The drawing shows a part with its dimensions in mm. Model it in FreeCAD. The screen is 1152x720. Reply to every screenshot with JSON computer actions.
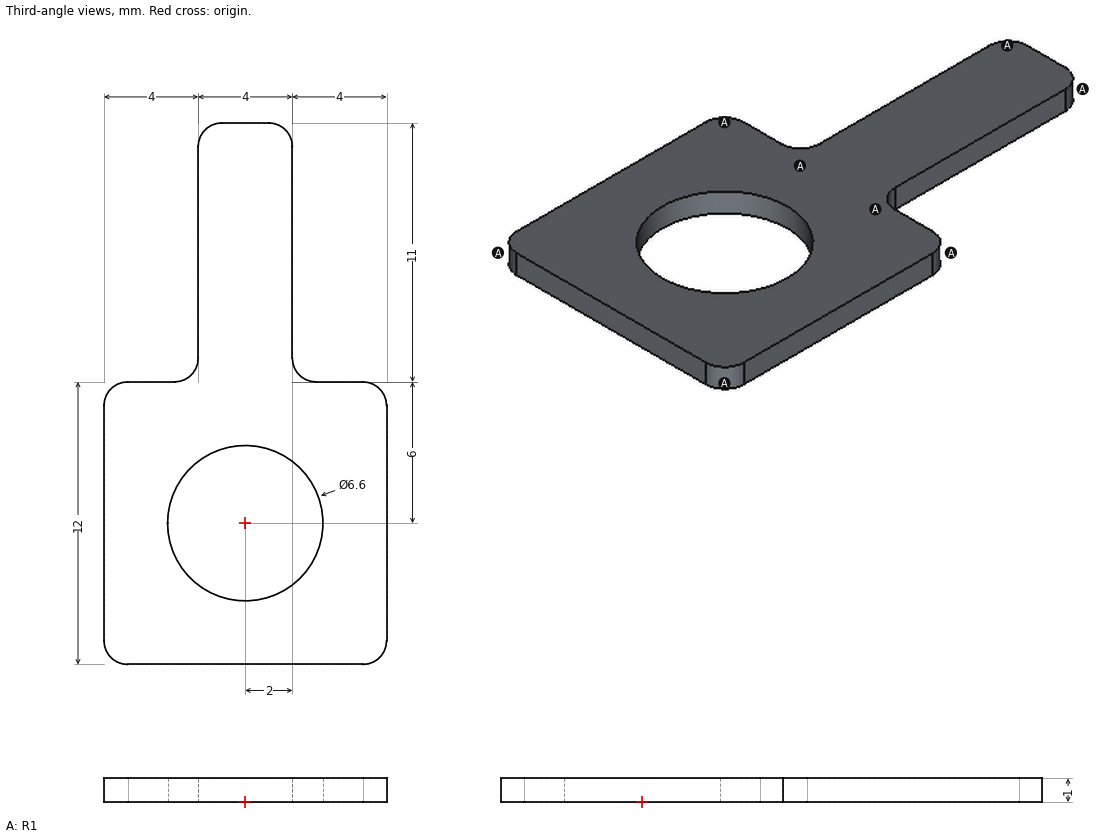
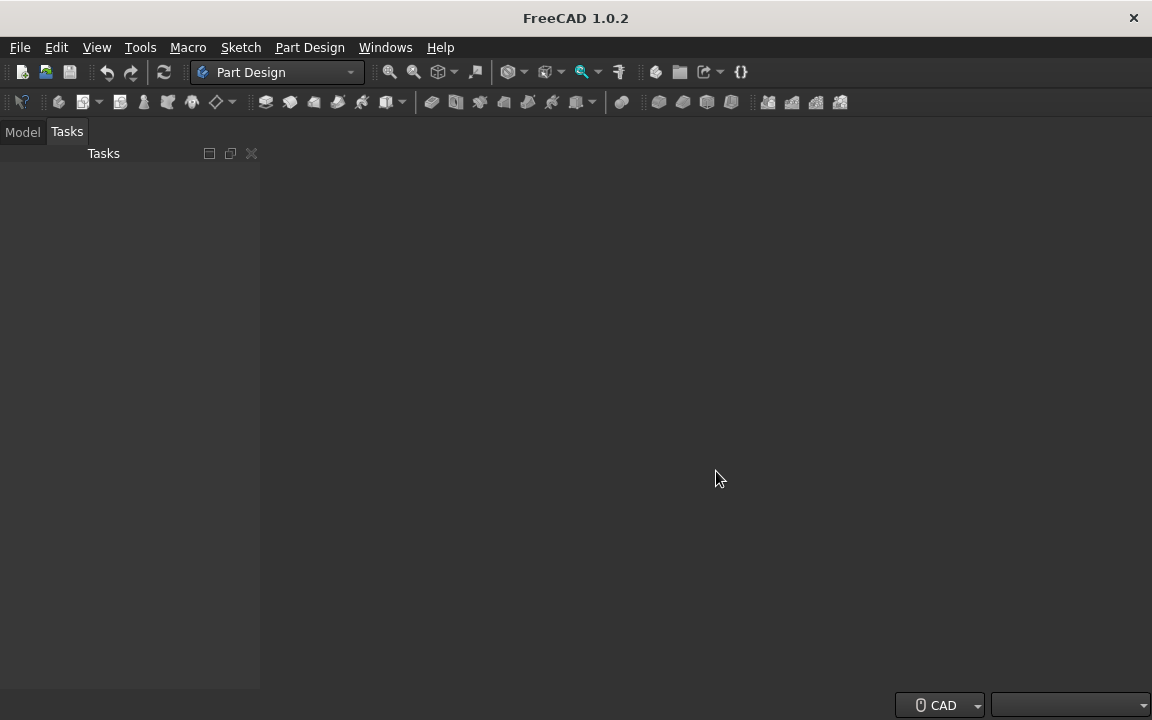
{"action": "left_click", "coordinate": [22, 72]}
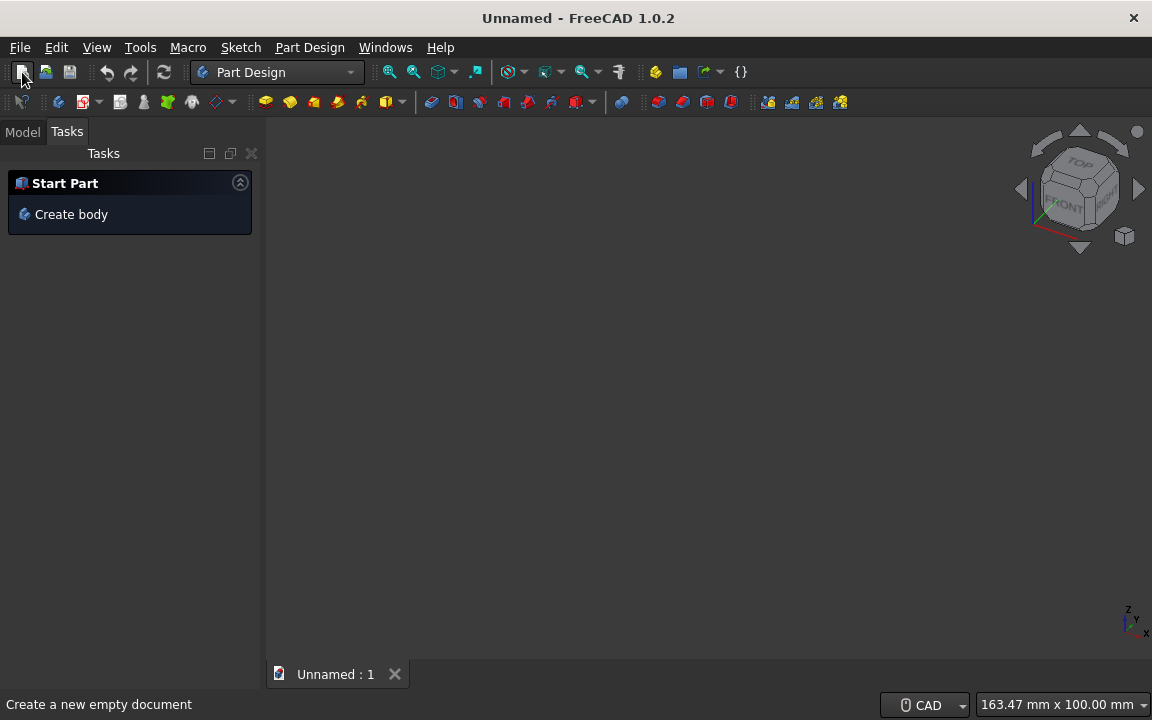
{"action": "left_click", "coordinate": [84, 102]}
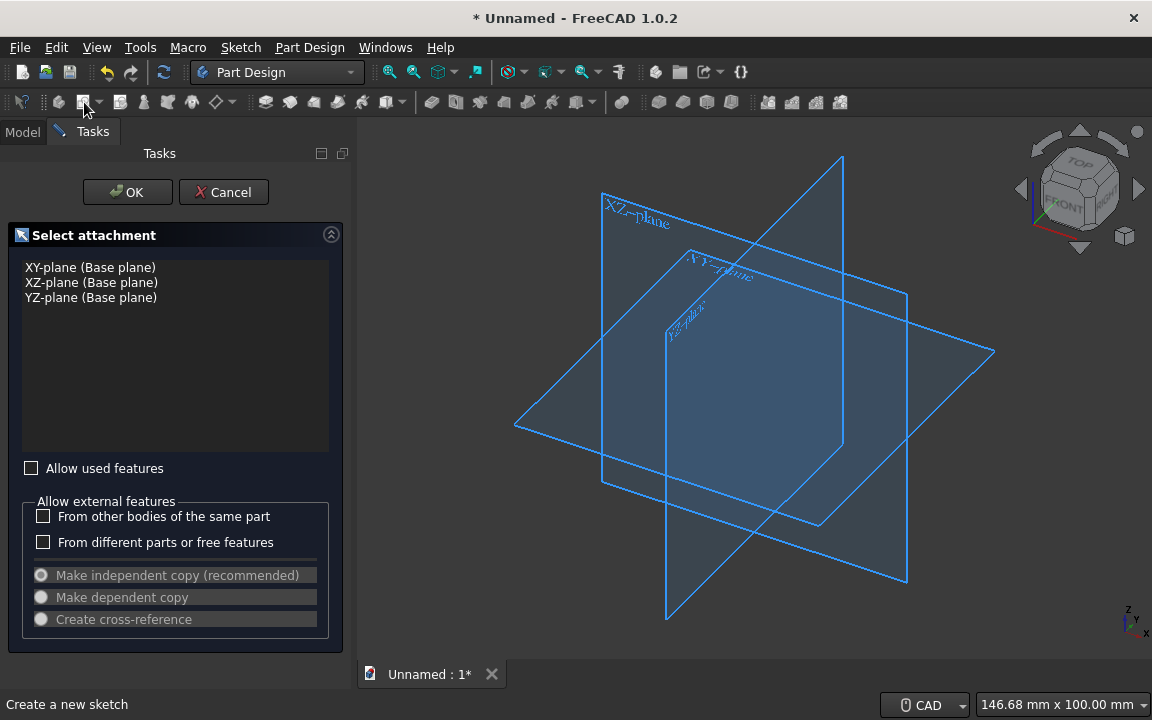
{"action": "left_click", "coordinate": [82, 268]}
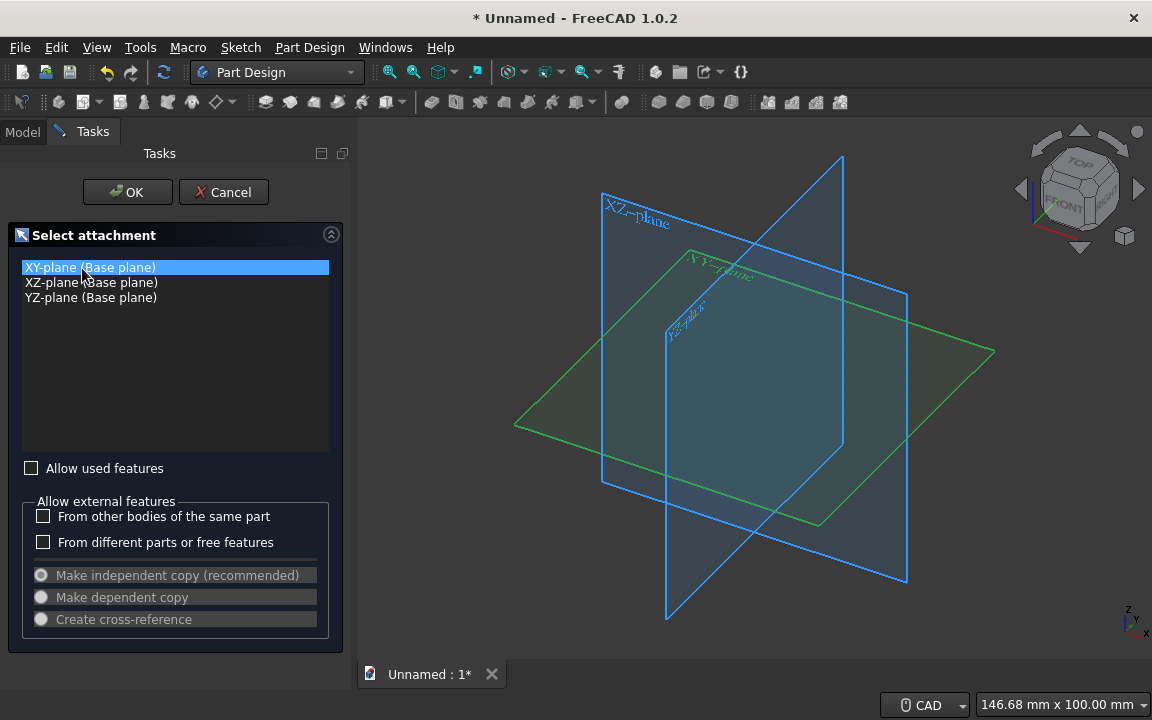
{"action": "left_click", "coordinate": [128, 192]}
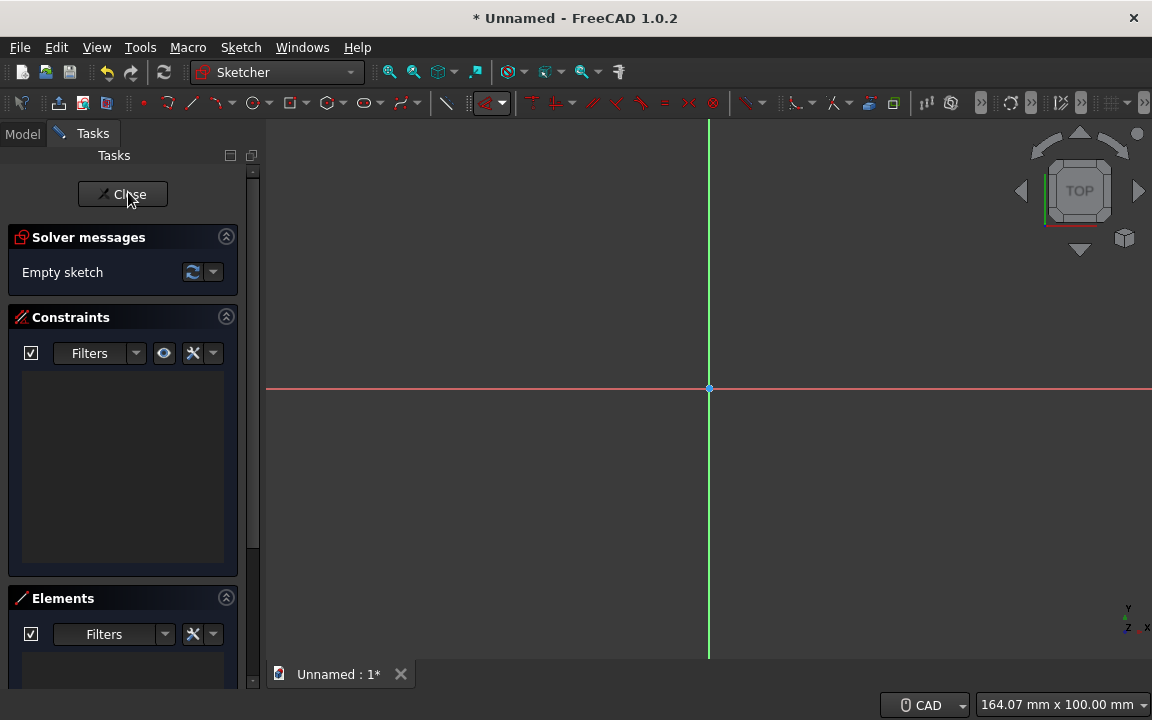
{"action": "scroll", "coordinate": [749, 342], "scroll_direction": "up", "scroll_amount": 5}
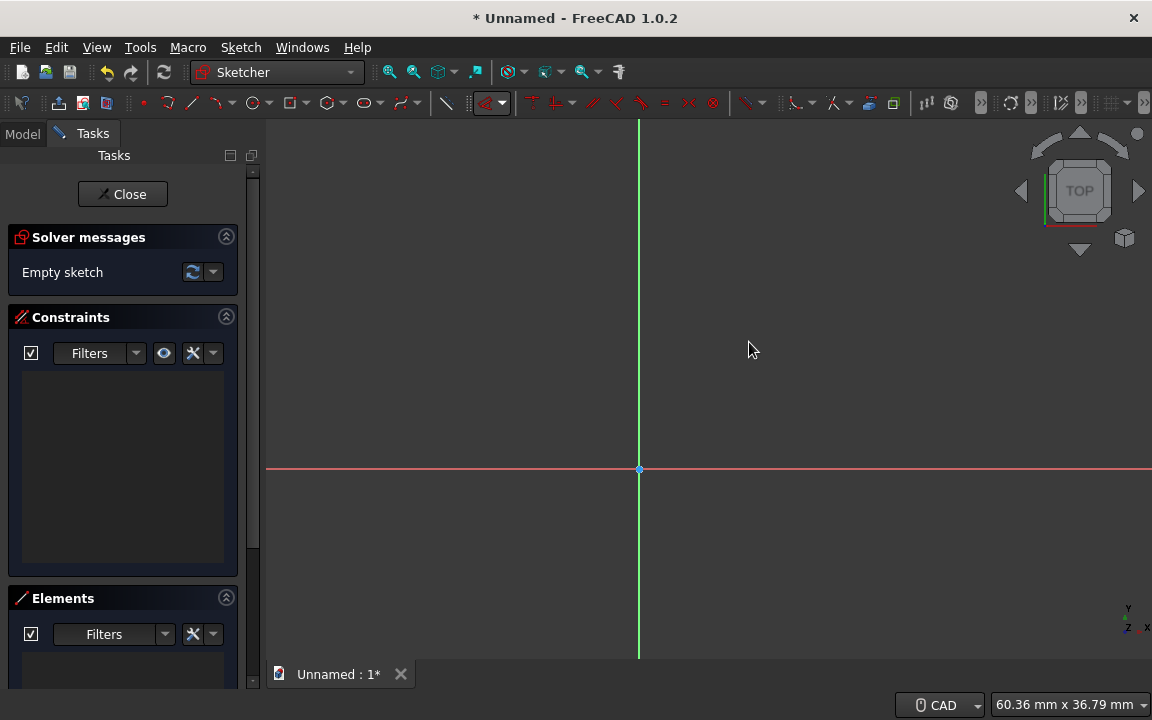
{"action": "key", "text": "g m"}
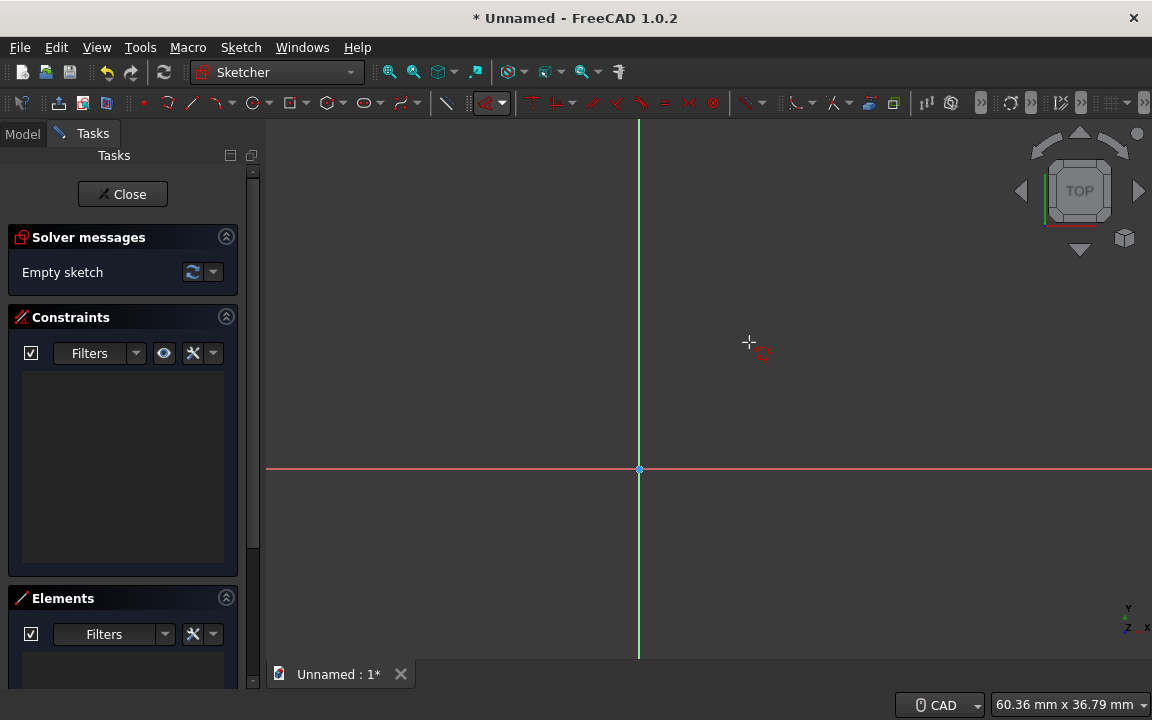
{"action": "left_click", "coordinate": [669, 381]}
{"action": "left_click", "coordinate": [669, 220]}
{"action": "left_click", "coordinate": [610, 220]}
{"action": "left_click", "coordinate": [610, 381]}
{"action": "left_click", "coordinate": [551, 381]}
{"action": "left_click", "coordinate": [551, 557]}
{"action": "left_click", "coordinate": [727, 557]}
{"action": "left_click", "coordinate": [727, 381]}
{"action": "left_click", "coordinate": [669, 382]}
{"action": "key", "text": "Escape"}
{"action": "key", "text": "Escape"}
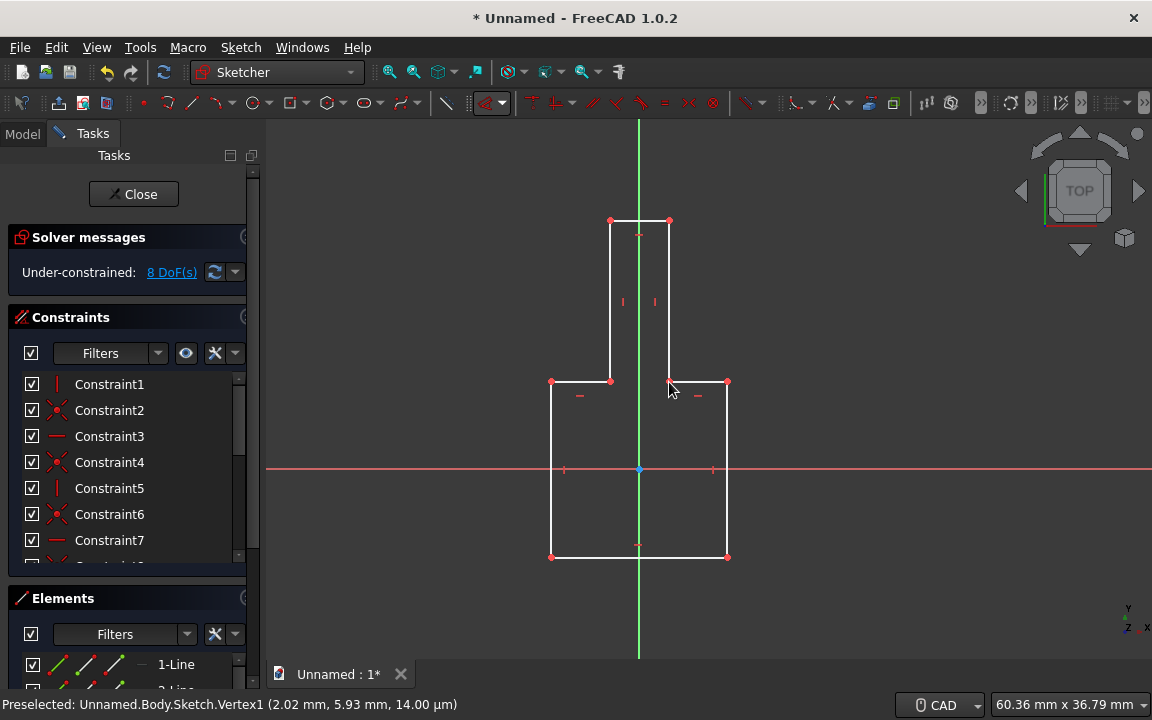
{"action": "left_click", "coordinate": [486, 104]}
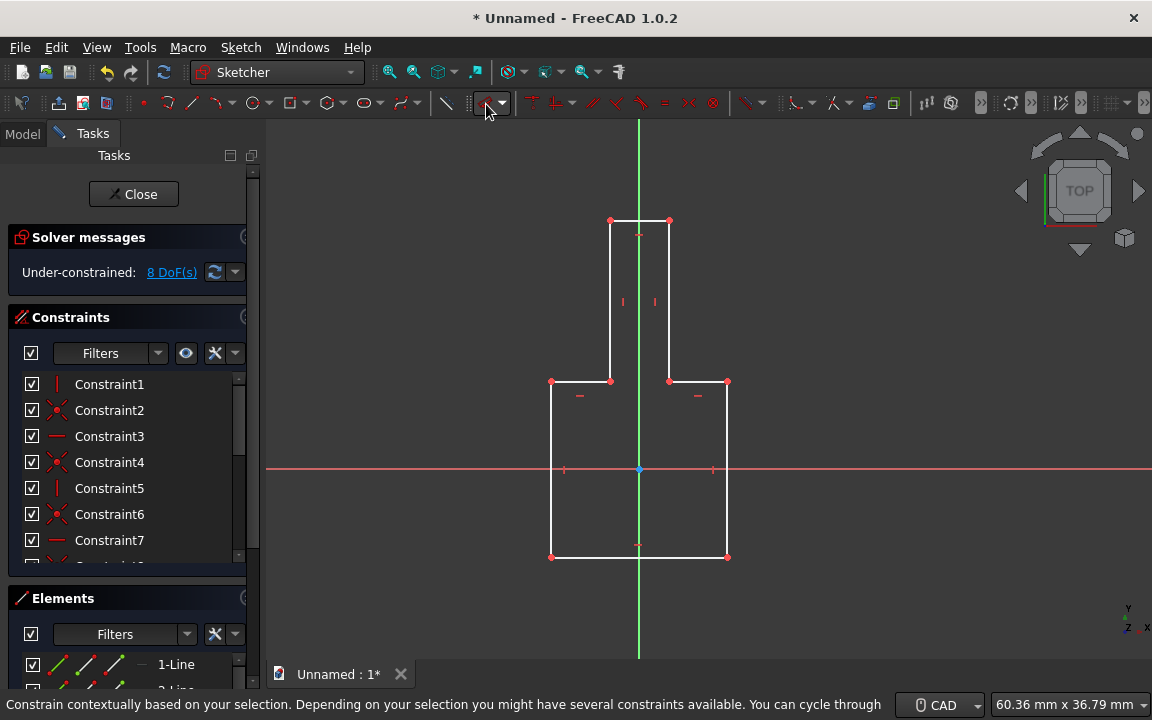
{"action": "left_click", "coordinate": [651, 221]}
{"action": "left_click", "coordinate": [626, 187]}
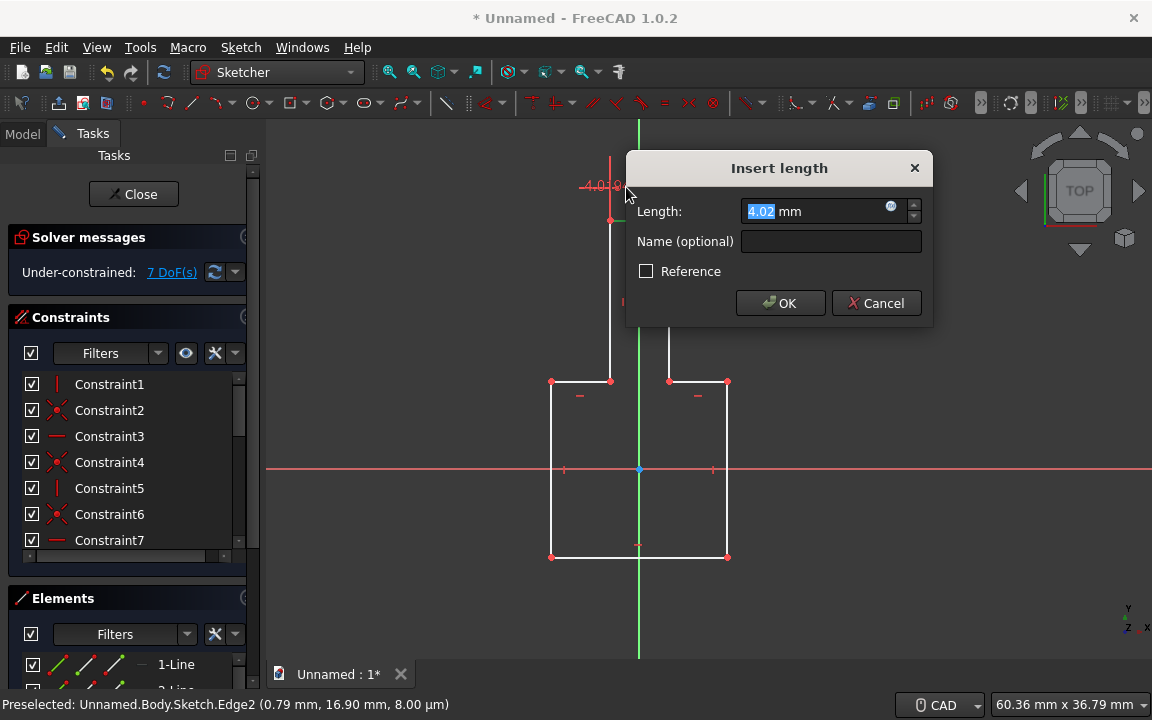
{"action": "type", "text": "4"}
{"action": "key", "text": "Return"}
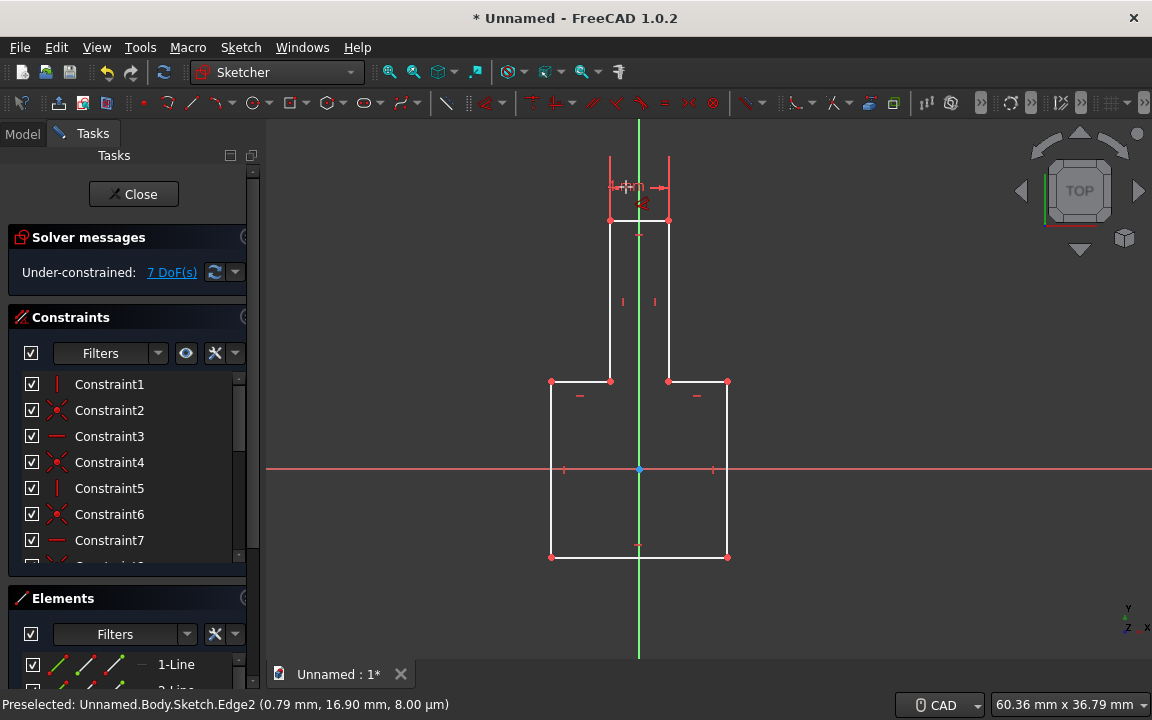
{"action": "left_click", "coordinate": [592, 382]}
{"action": "left_click", "coordinate": [580, 348]}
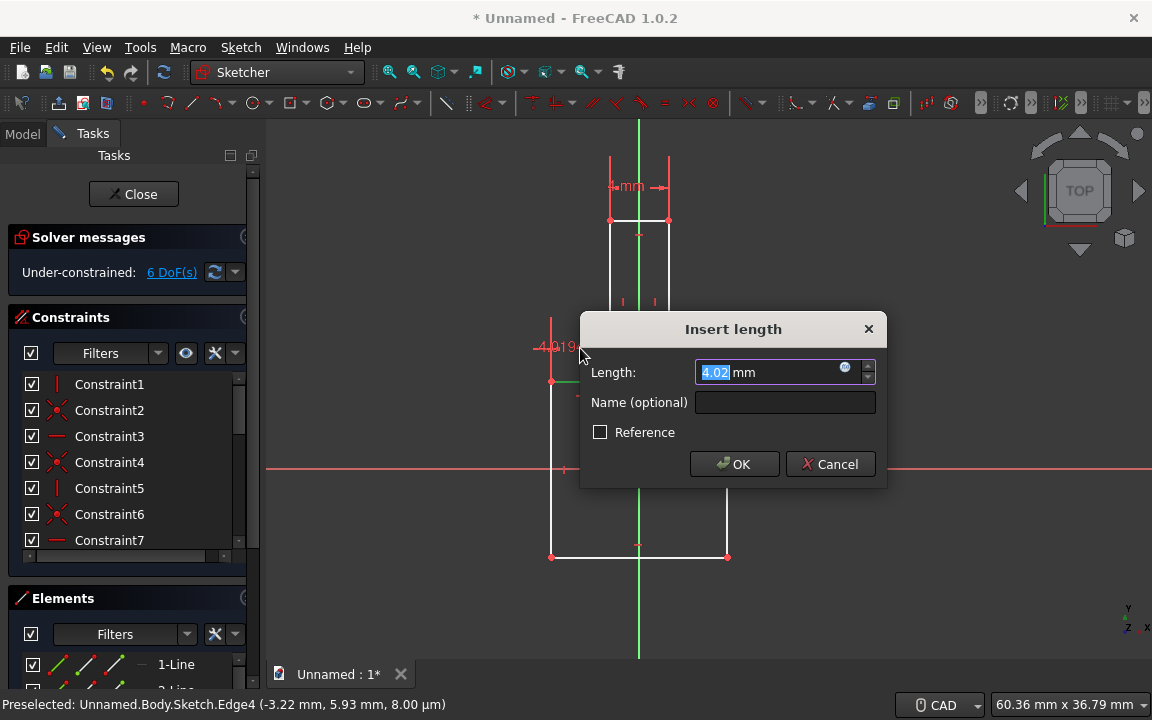
{"action": "type", "text": "4"}
{"action": "key", "text": "Return"}